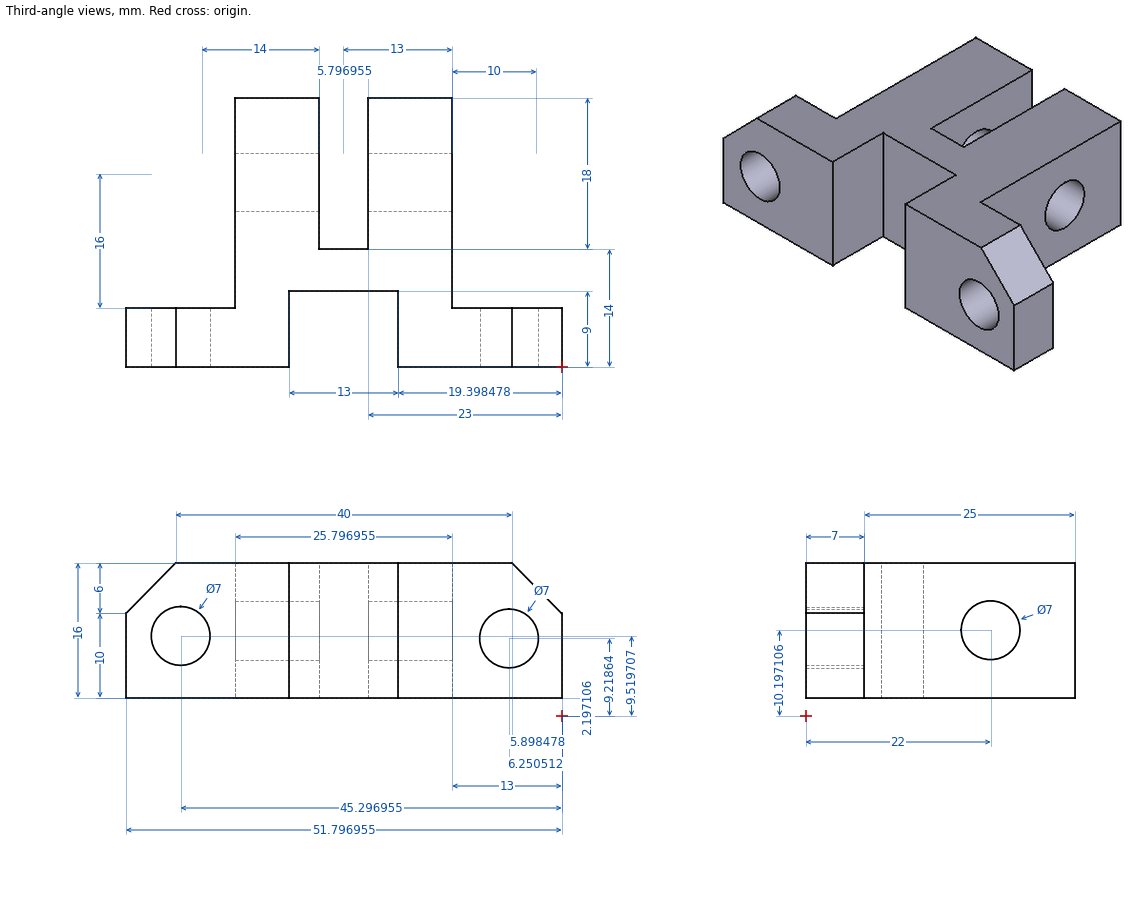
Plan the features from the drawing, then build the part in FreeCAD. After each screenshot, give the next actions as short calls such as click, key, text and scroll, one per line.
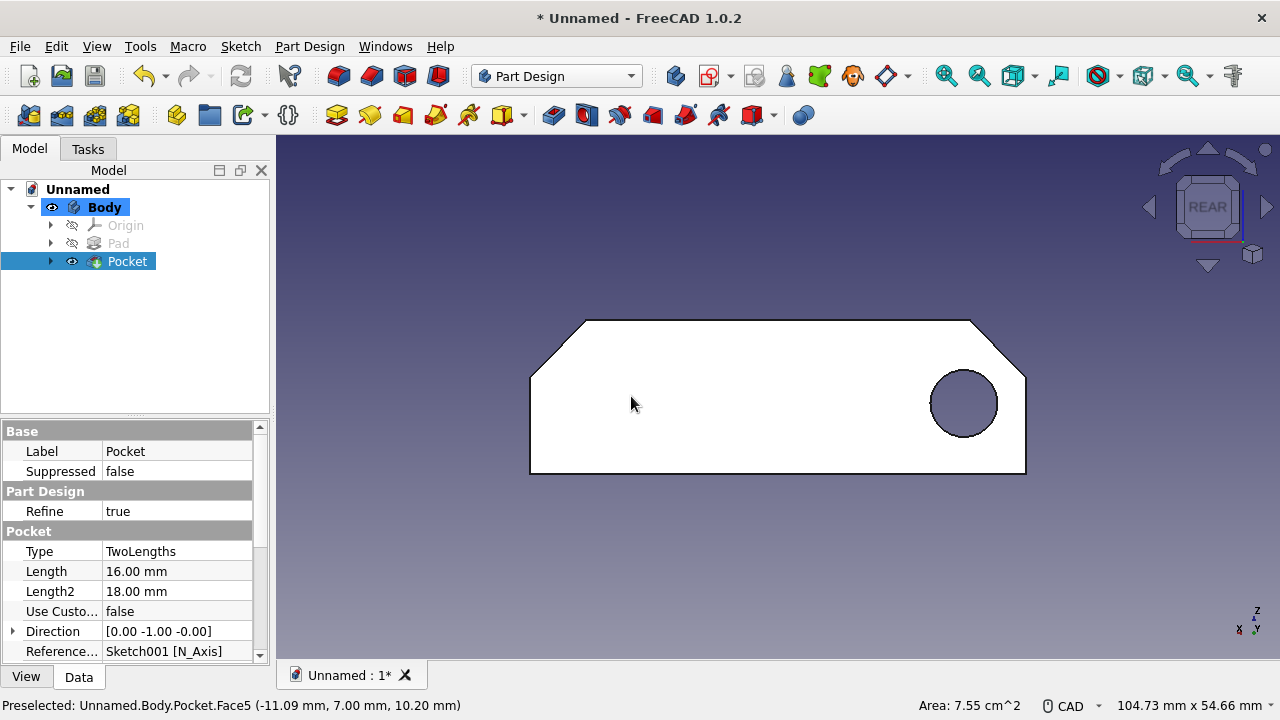
click(708, 76)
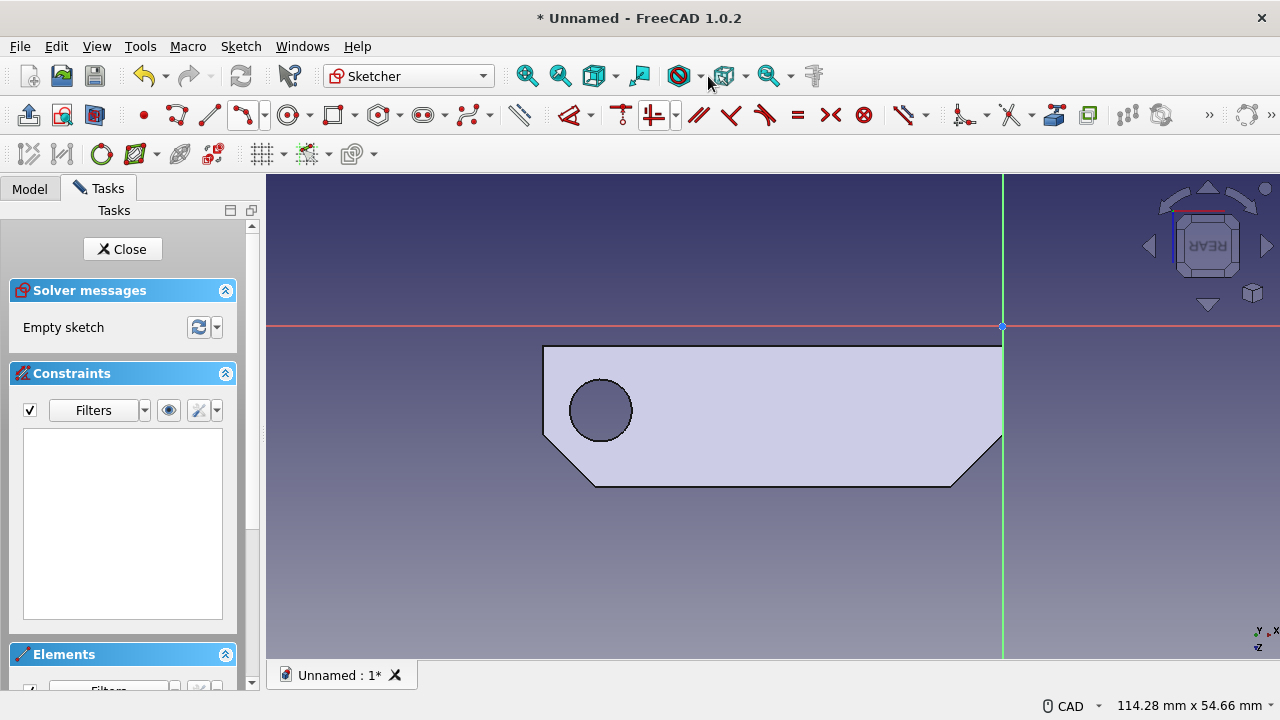
scroll(1108, 363, up, 5)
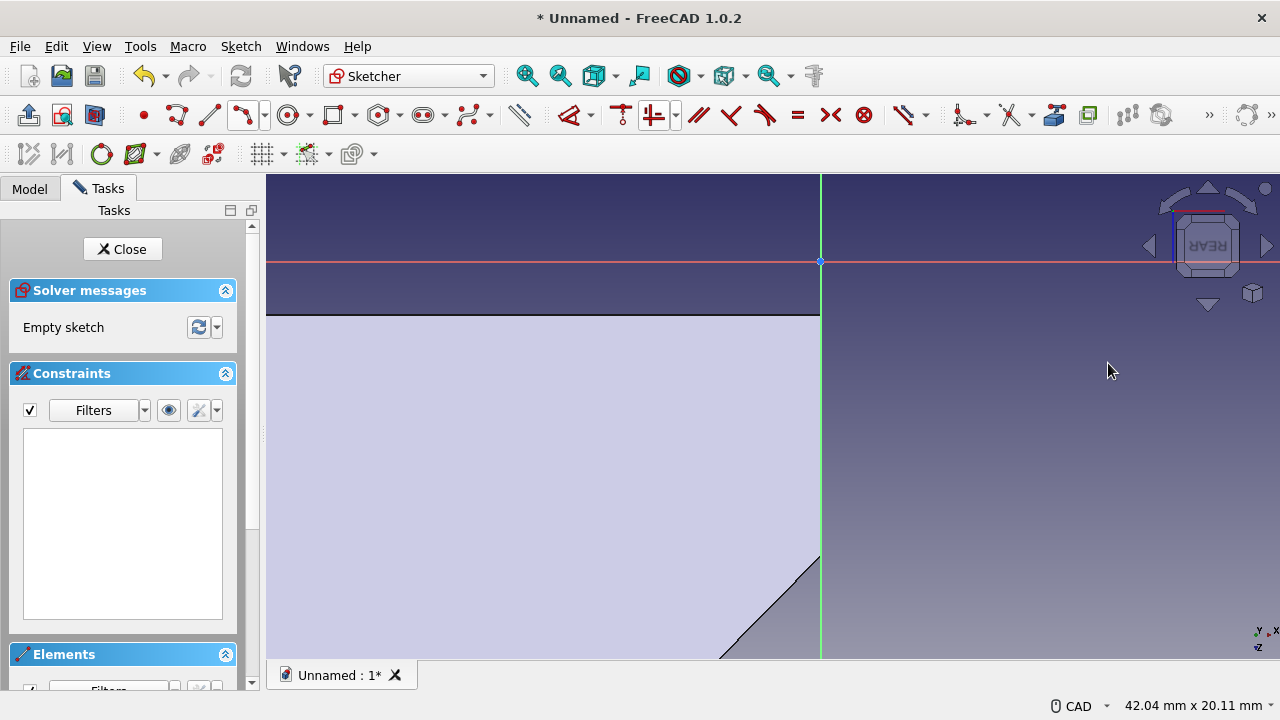
key(g)
key(c)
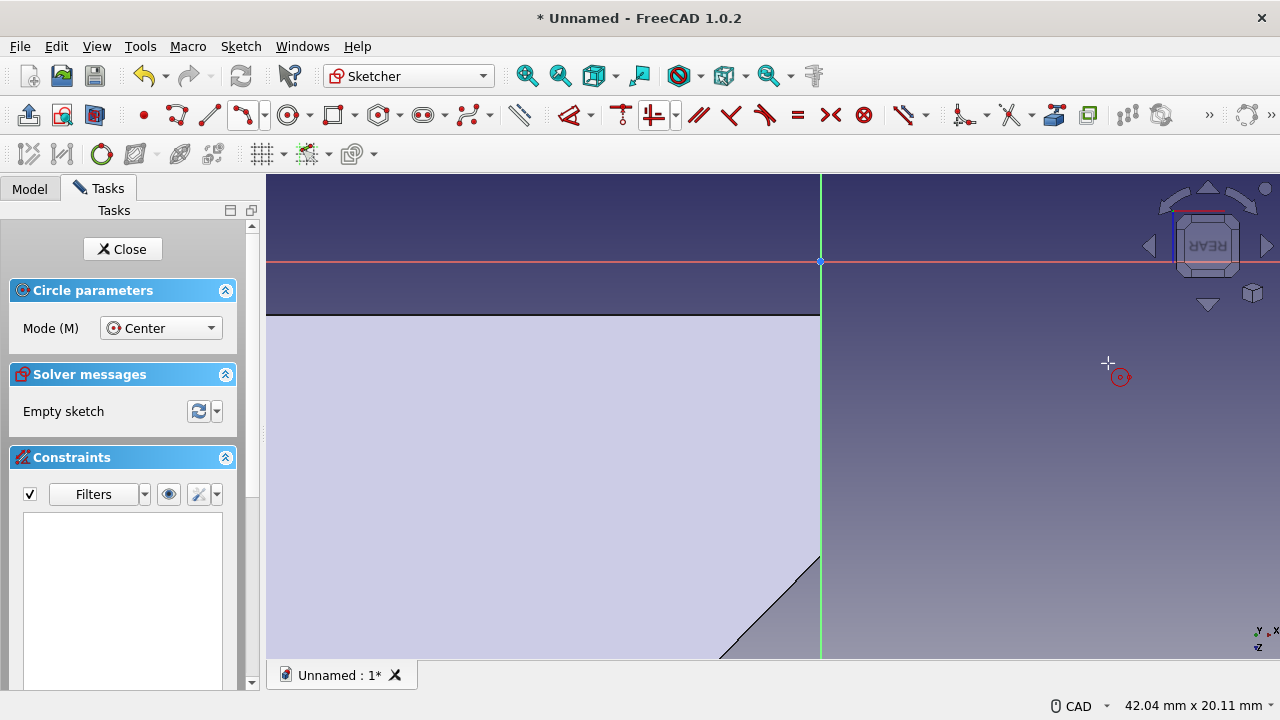
click(670, 484)
click(730, 424)
key(Escape)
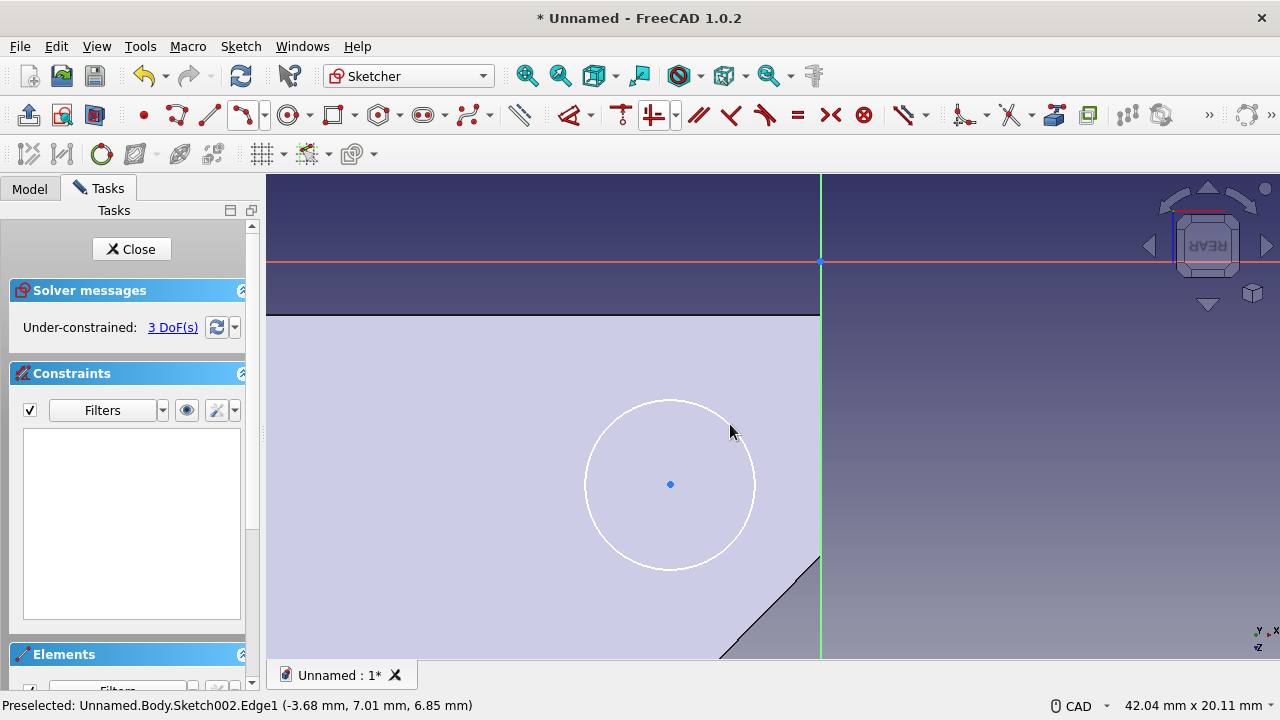
key(d)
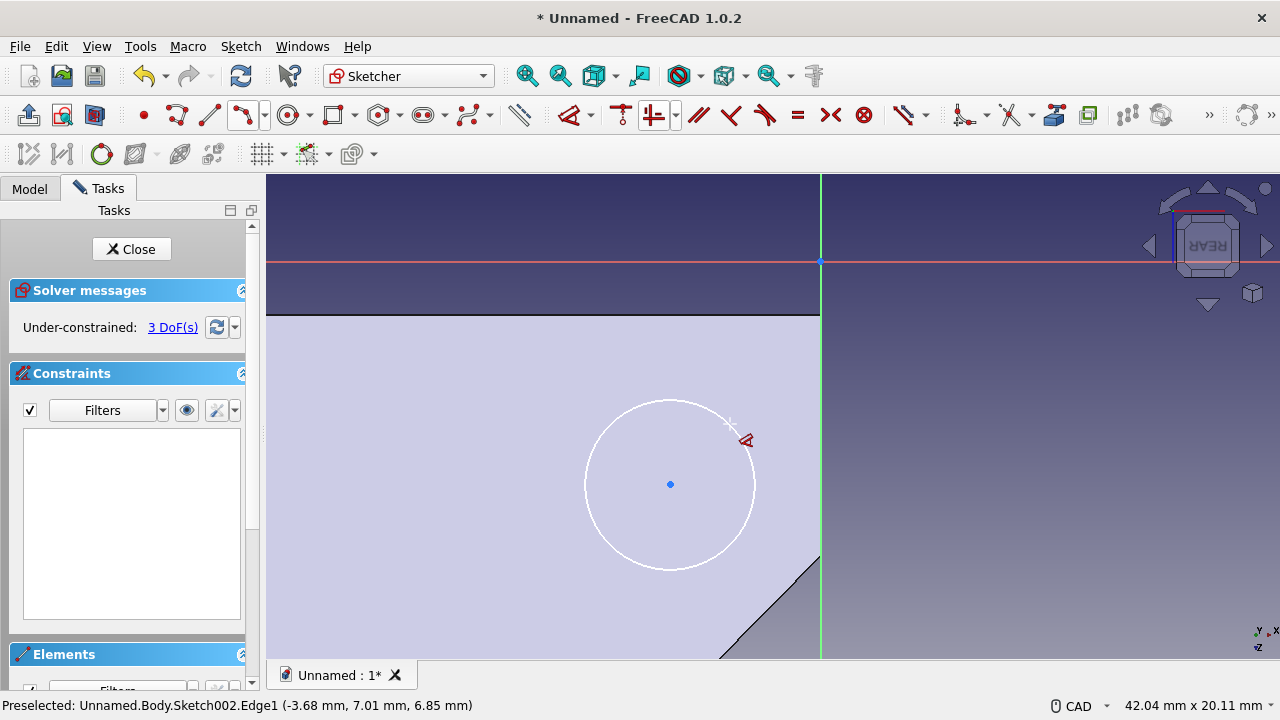
click(730, 425)
click(753, 402)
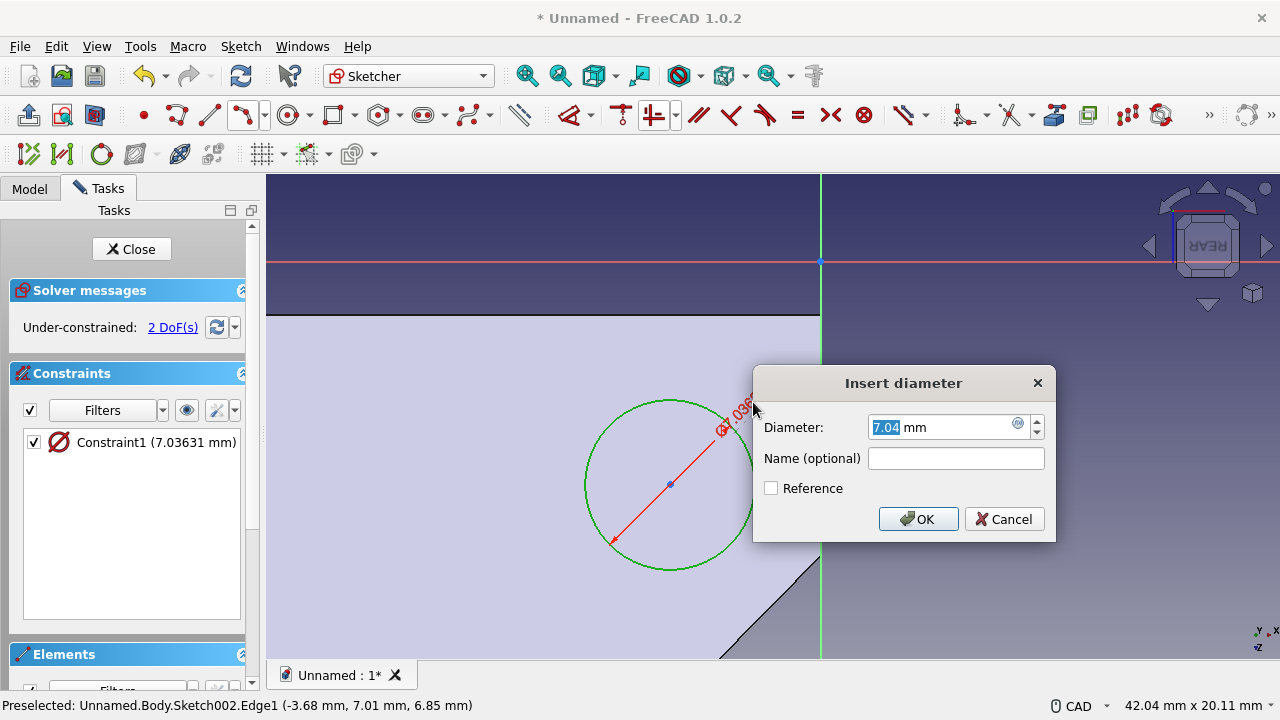
text(7)
key(Return)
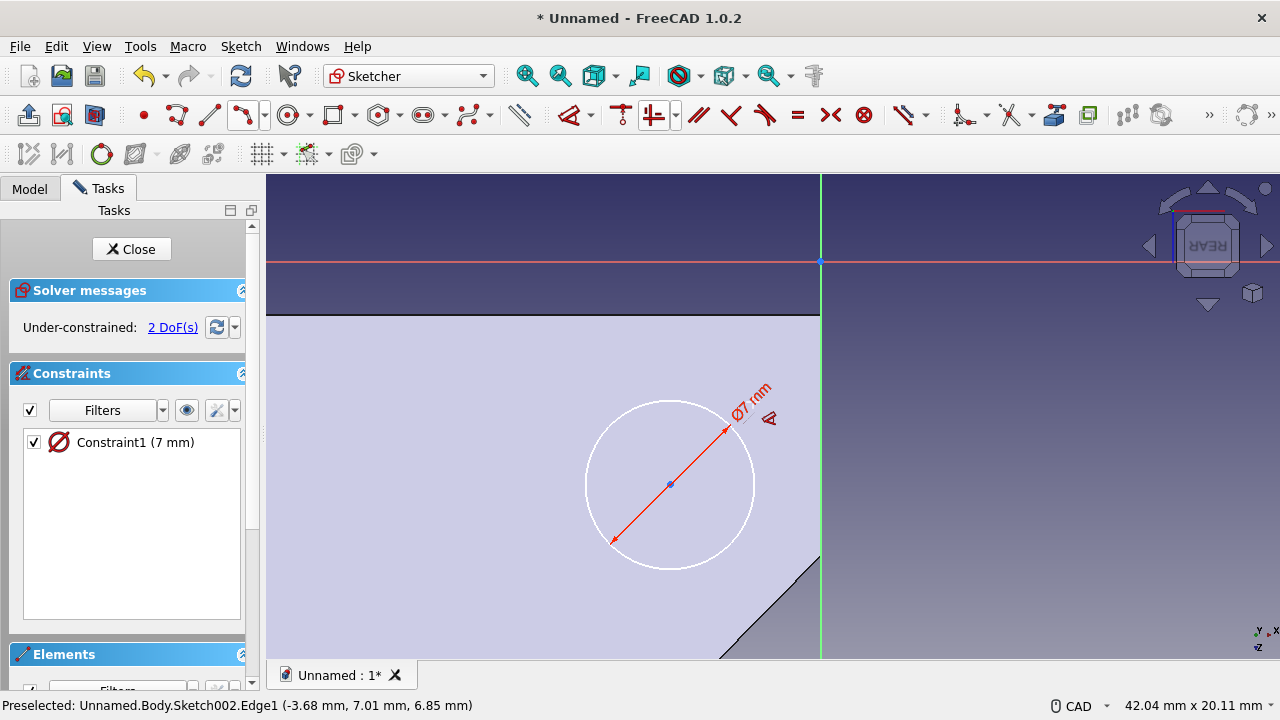
click(670, 485)
click(855, 373)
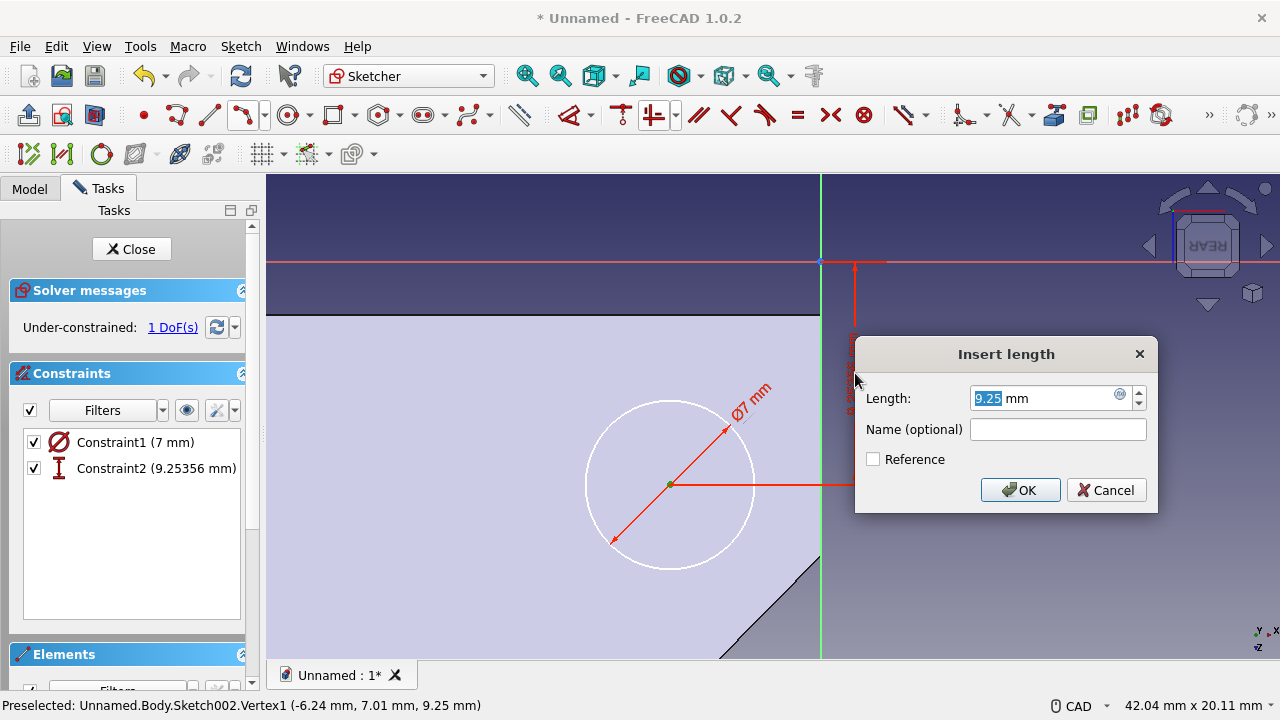
text(9.21864)
key(Return)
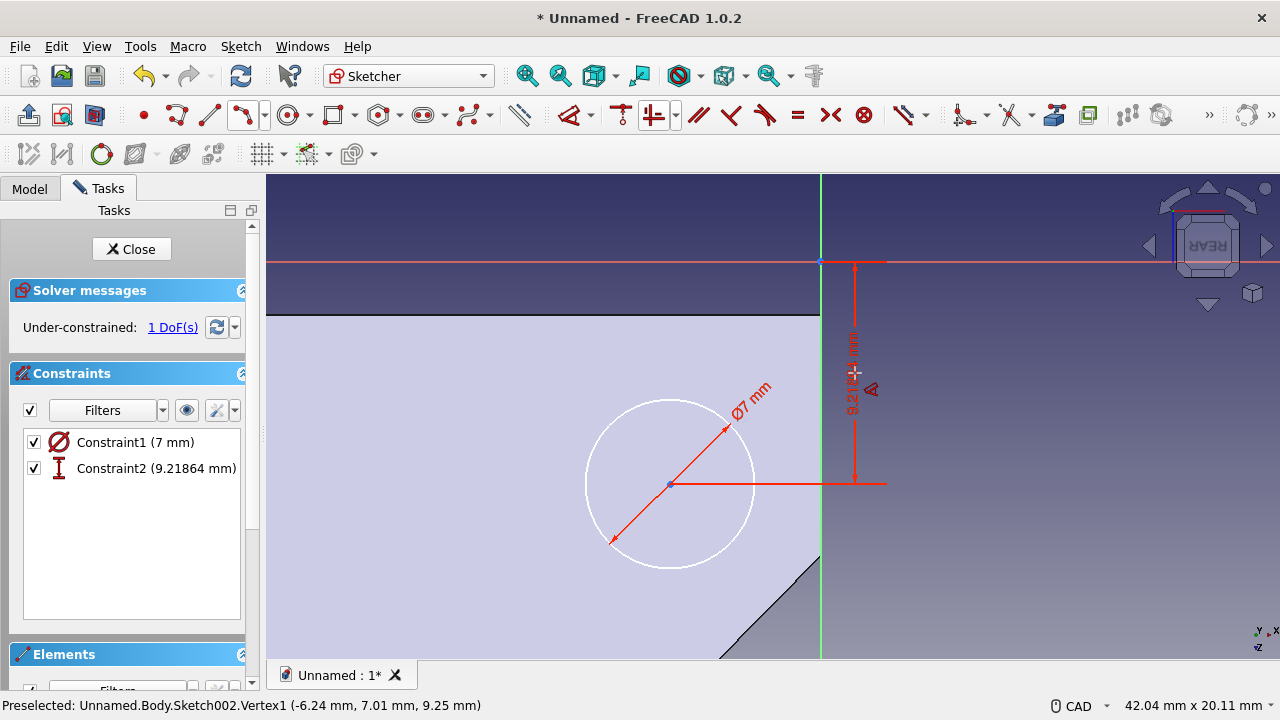
click(670, 484)
click(745, 228)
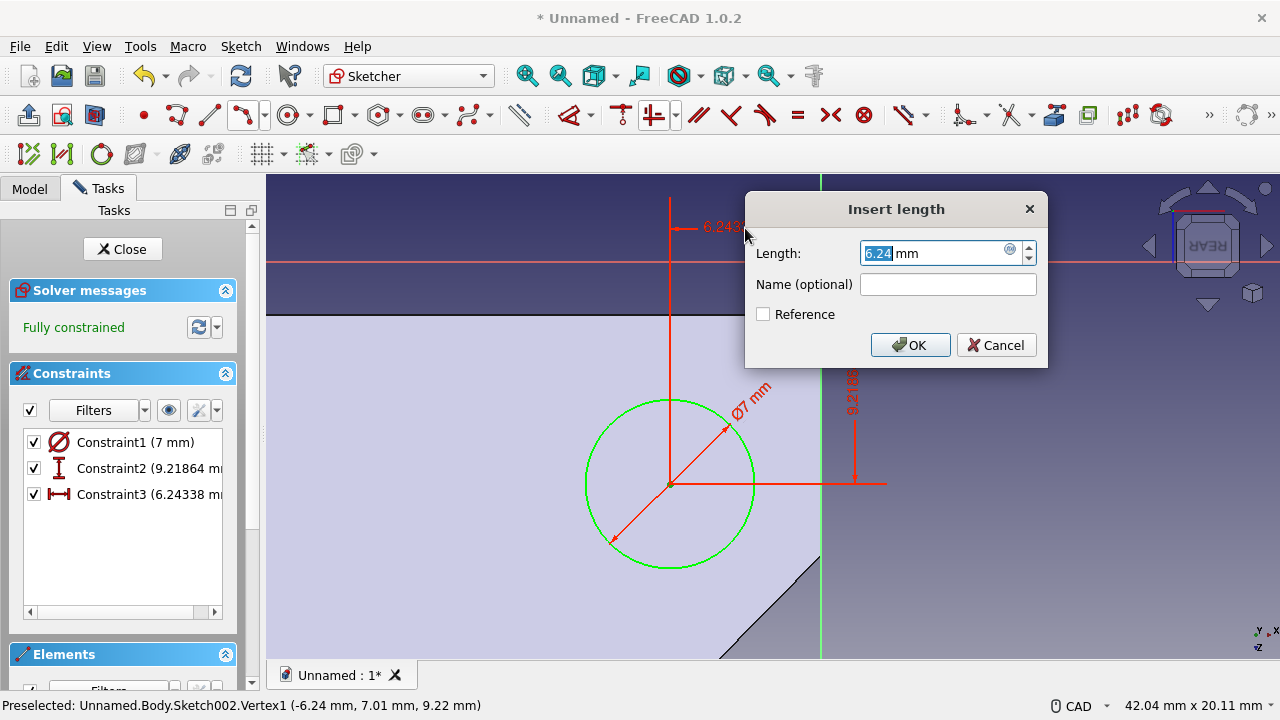
text(6.250512)
key(Return)
key(Escape)